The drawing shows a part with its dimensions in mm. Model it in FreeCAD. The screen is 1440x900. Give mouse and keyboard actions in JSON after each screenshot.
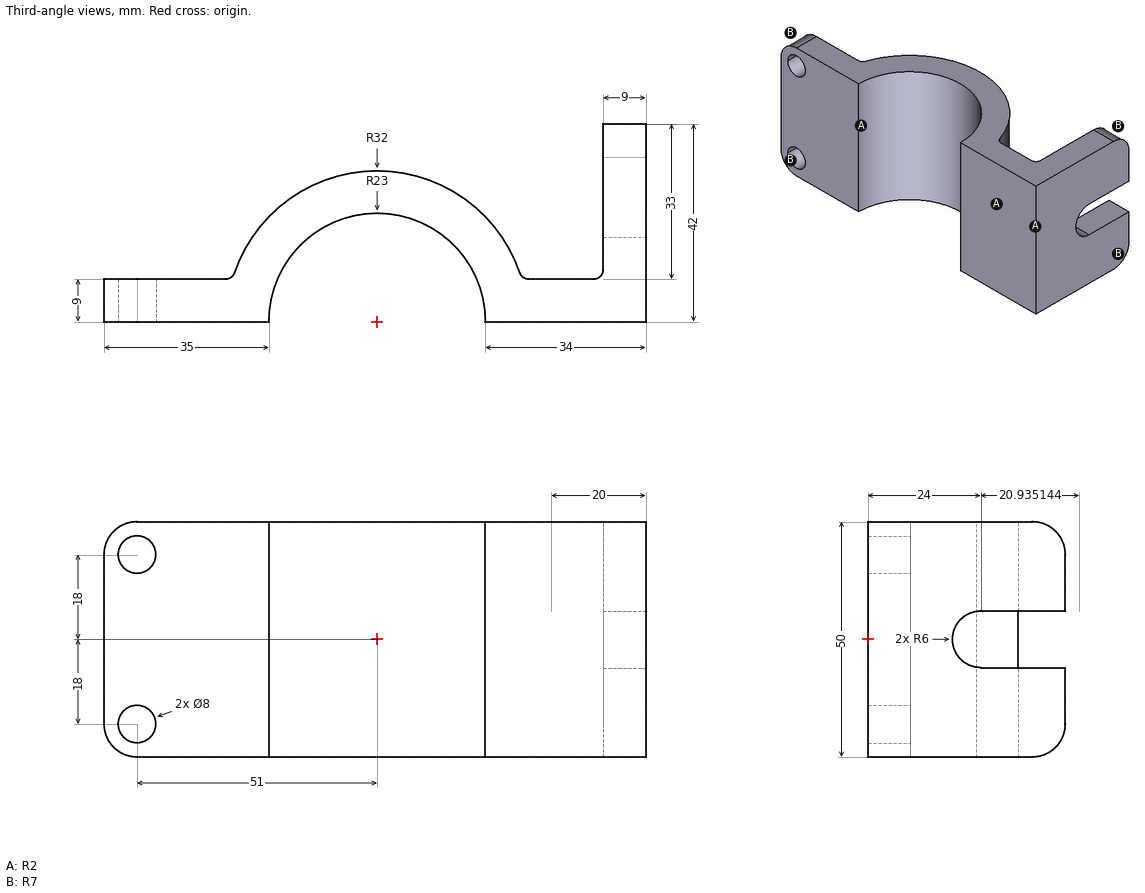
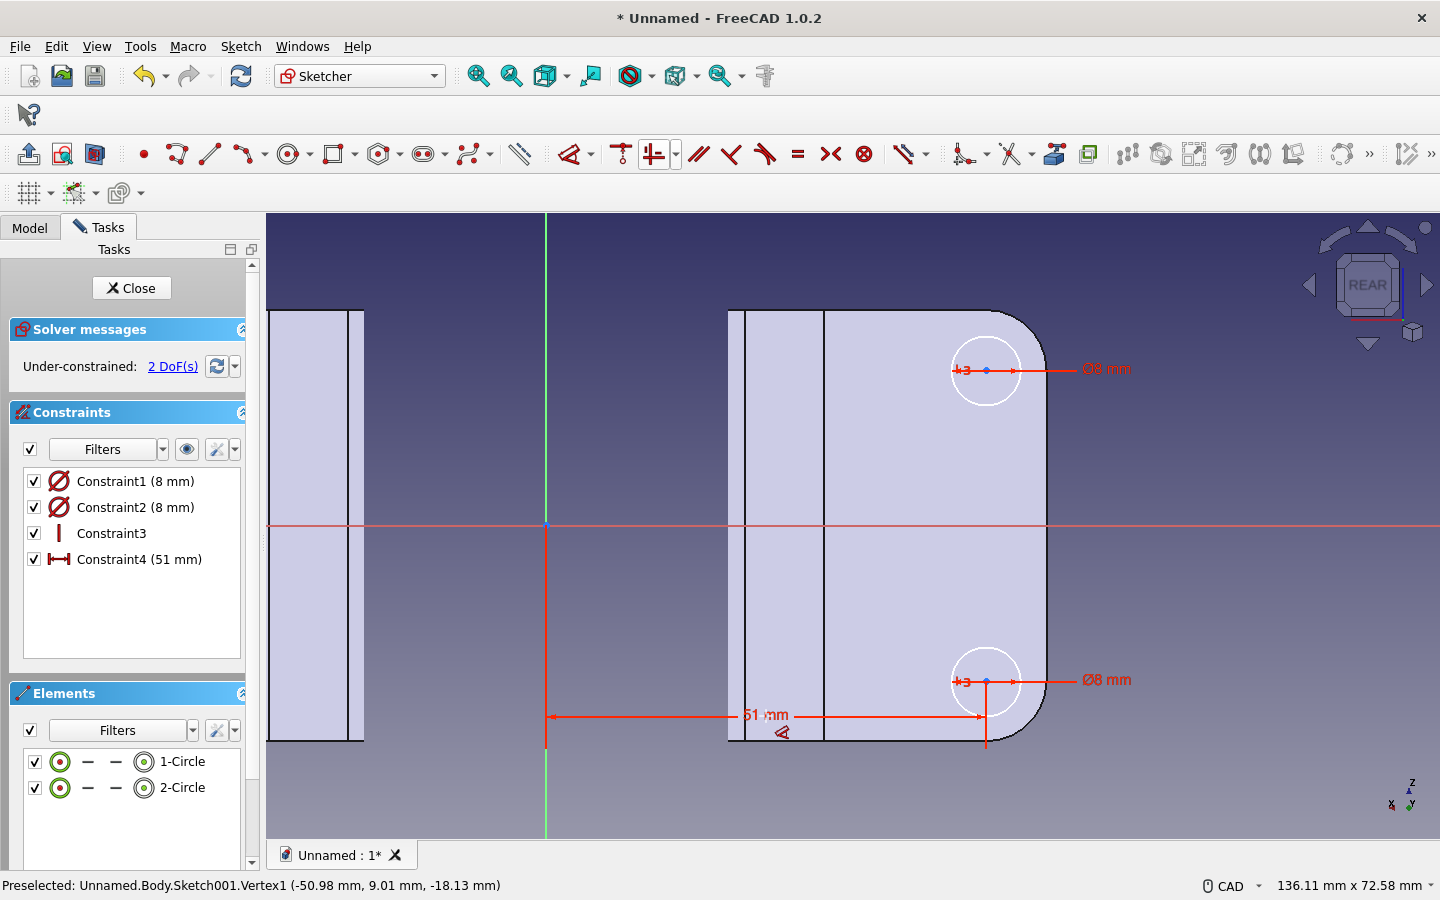
{"action": "left_click", "coordinate": [986, 682]}
{"action": "left_click", "coordinate": [512, 604]}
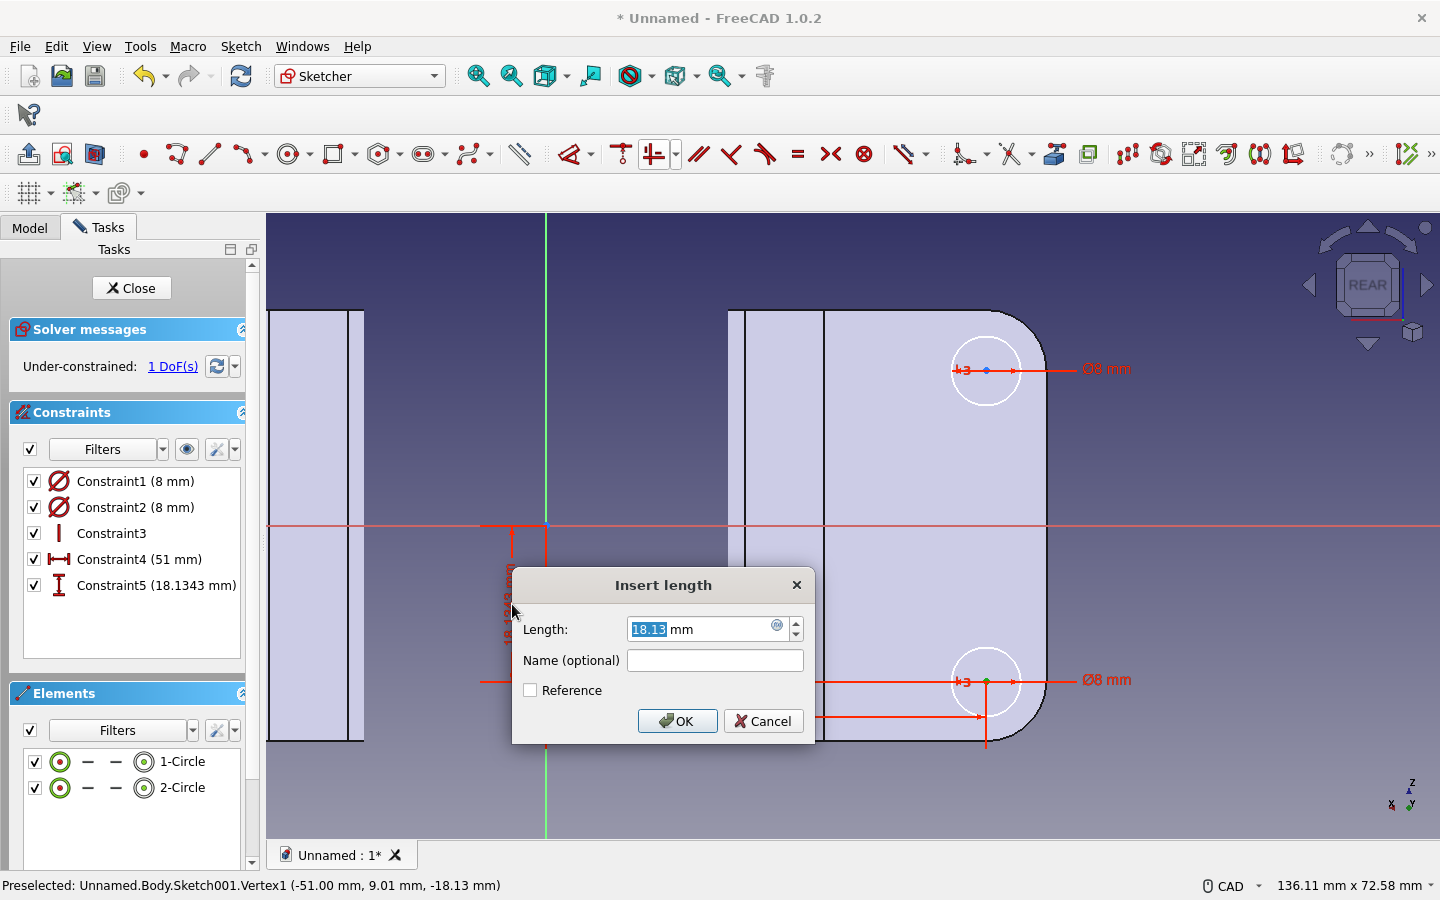
{"action": "type", "text": "18"}
{"action": "key", "text": "Return"}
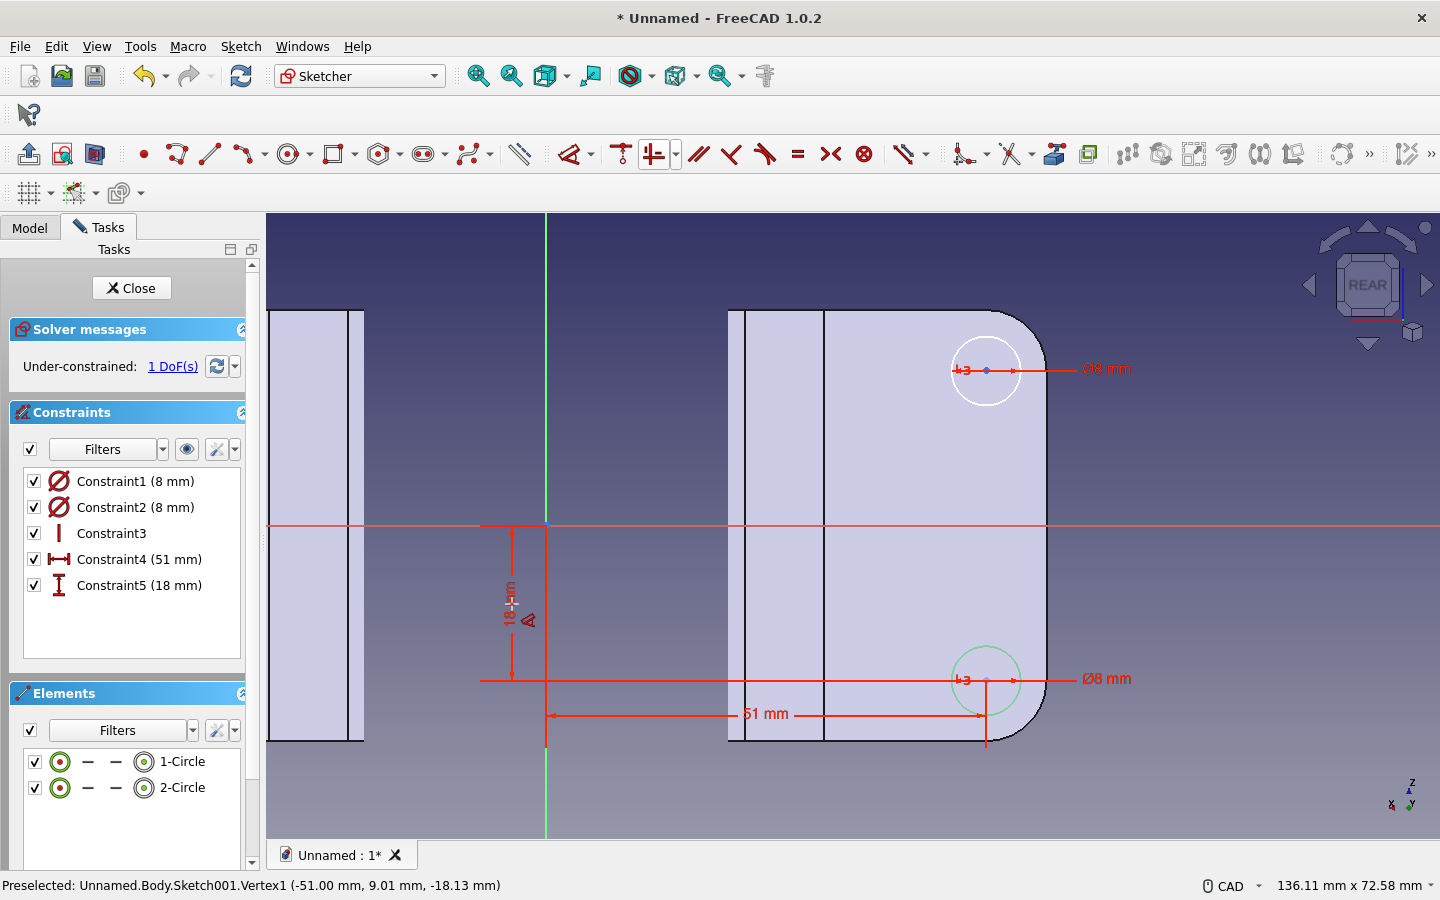
{"action": "left_click", "coordinate": [986, 371]}
{"action": "left_click", "coordinate": [512, 448]}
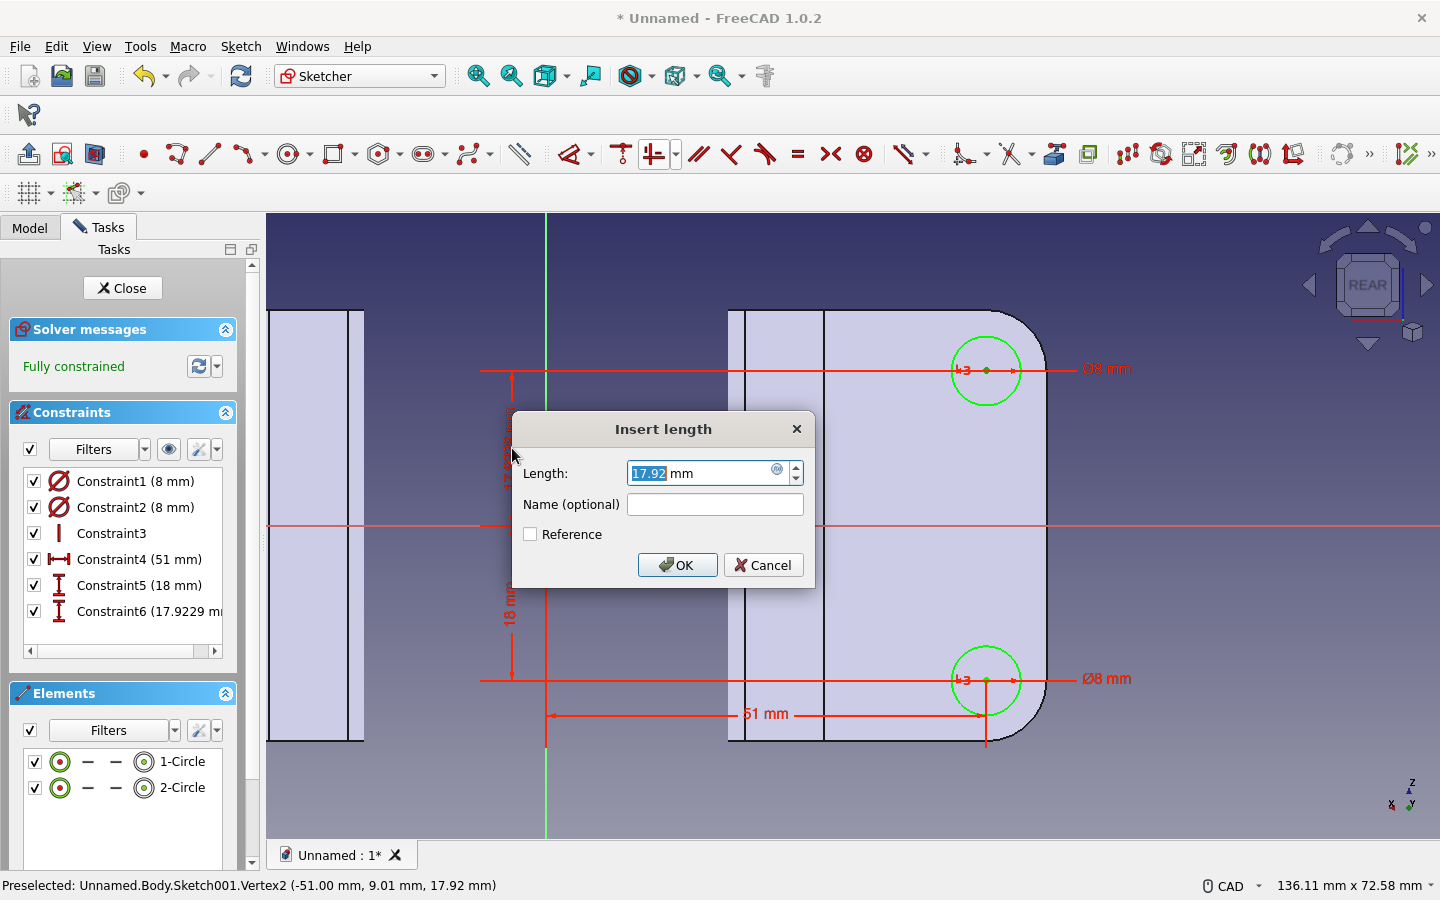
{"action": "type", "text": "18"}
{"action": "key", "text": "Return"}
{"action": "key", "text": "Escape"}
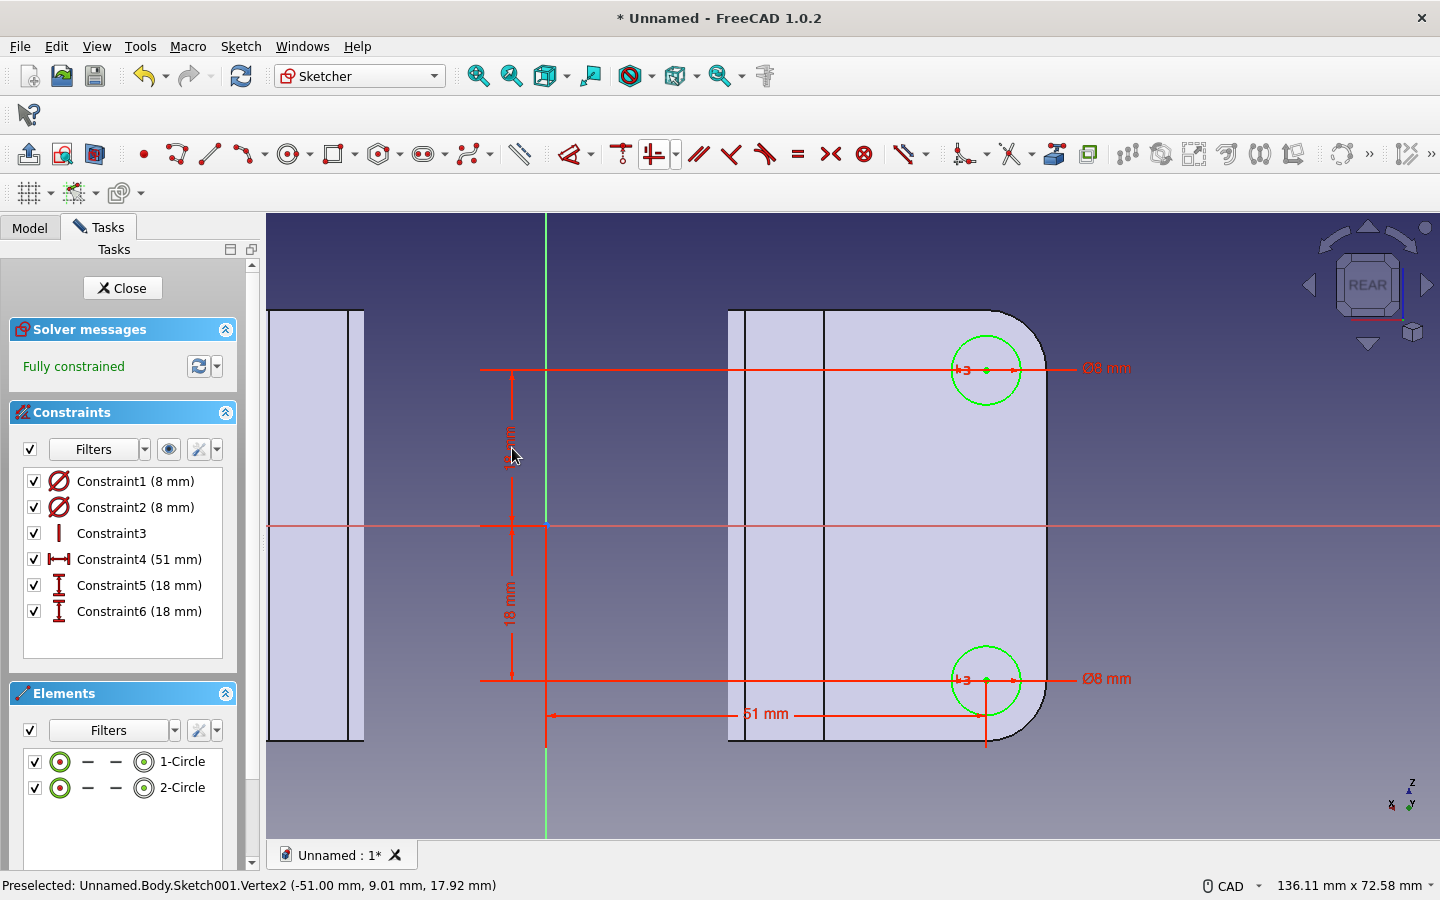
{"action": "left_click", "coordinate": [123, 288]}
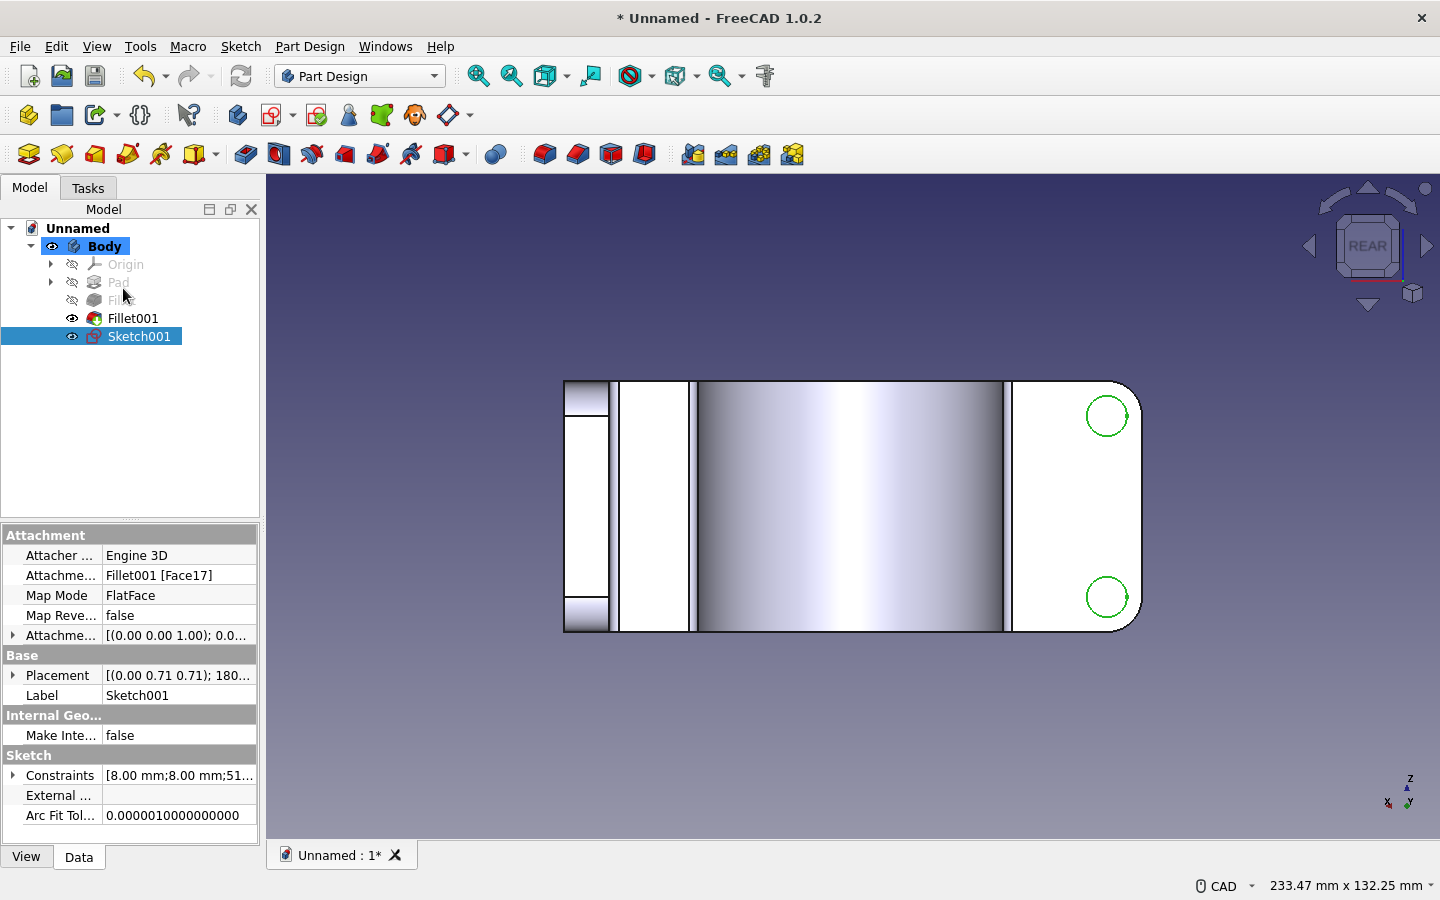
{"action": "left_click", "coordinate": [246, 154]}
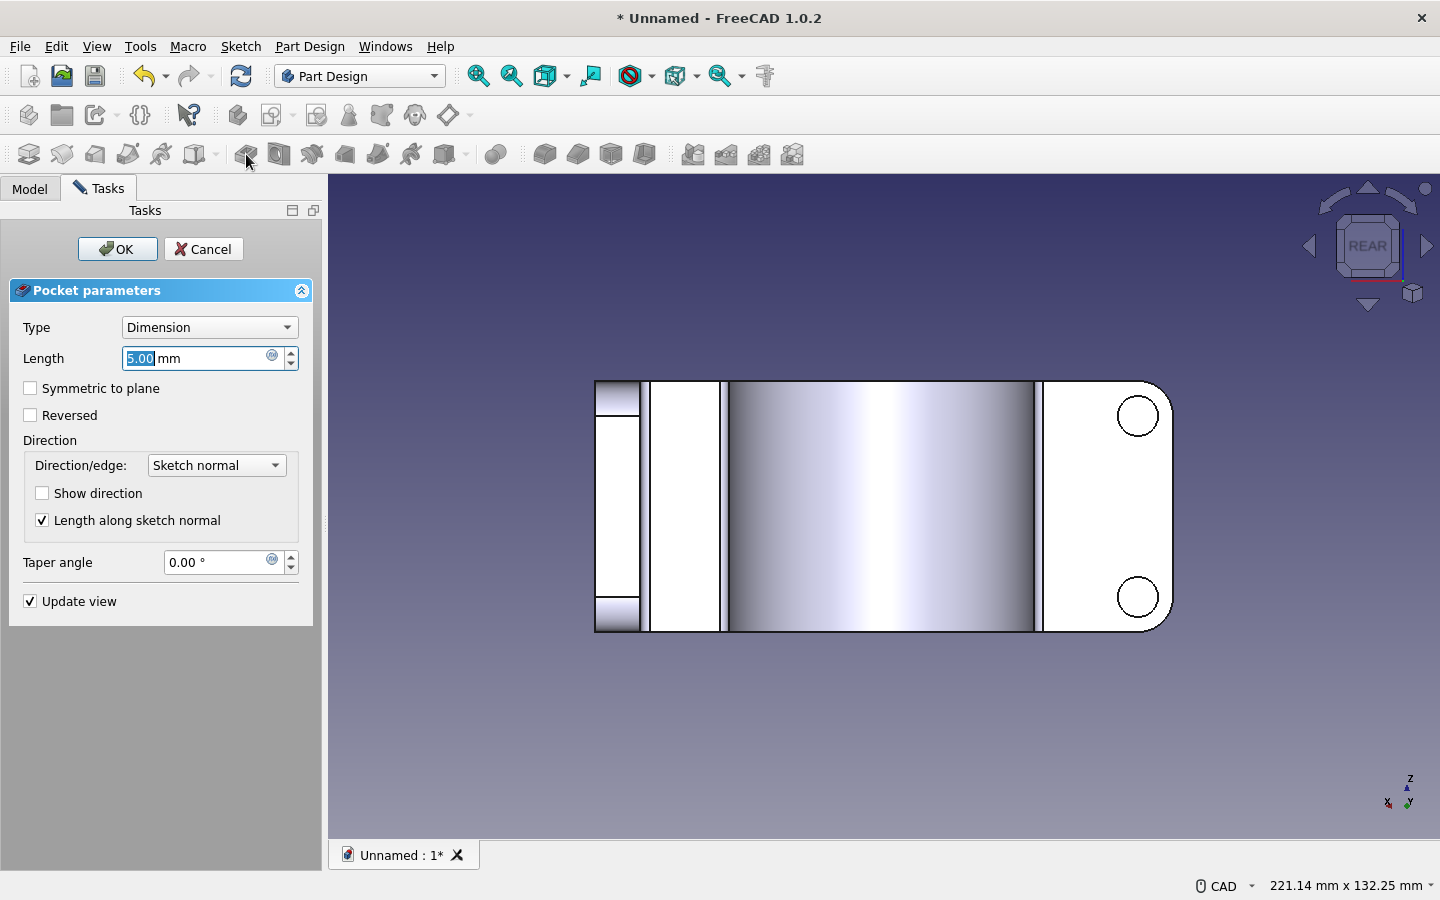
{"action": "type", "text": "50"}
{"action": "key", "text": "Tab"}